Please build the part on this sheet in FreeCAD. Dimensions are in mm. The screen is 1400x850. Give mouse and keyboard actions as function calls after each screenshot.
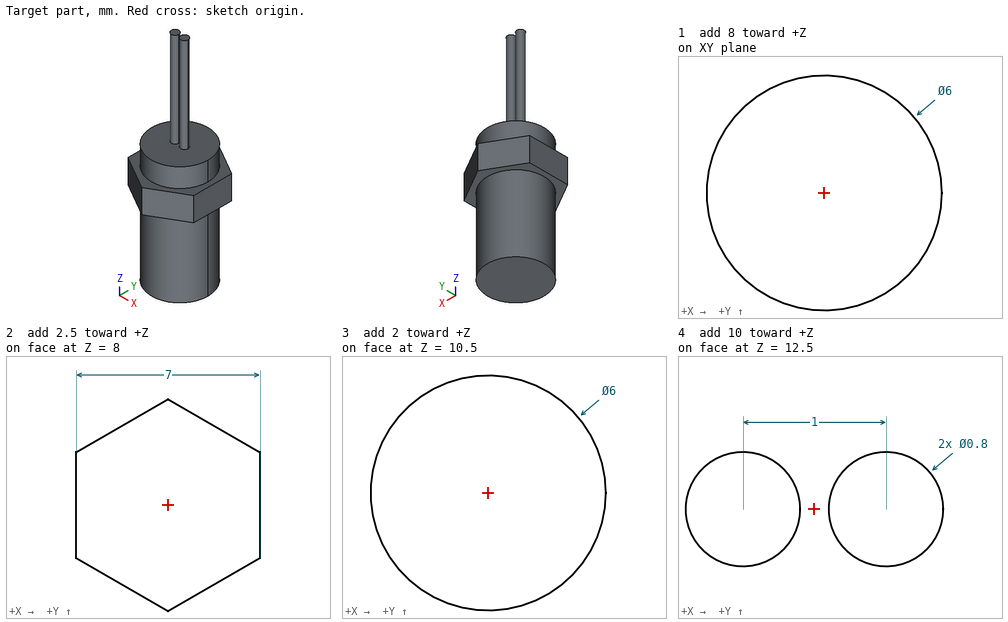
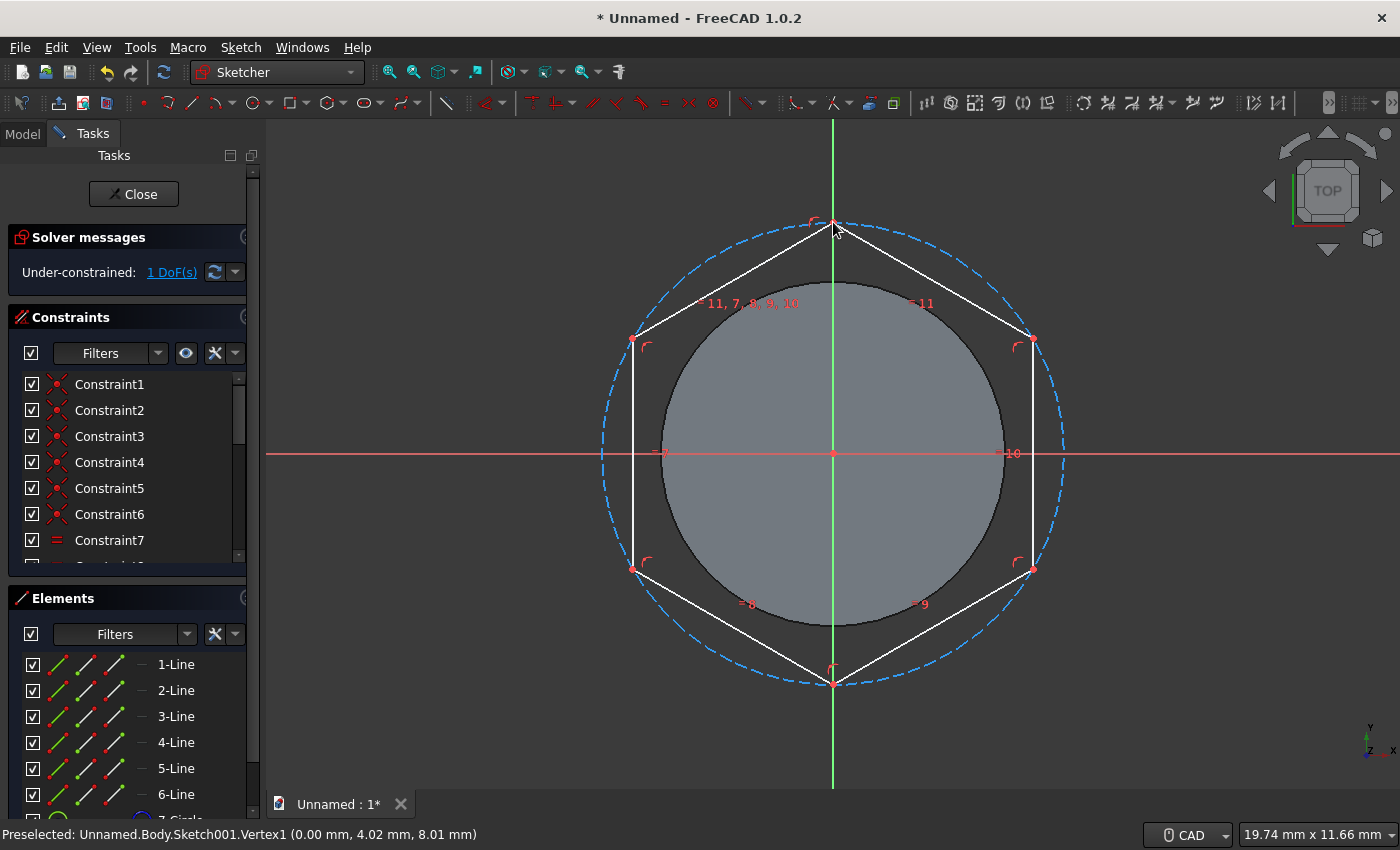
click(633, 339)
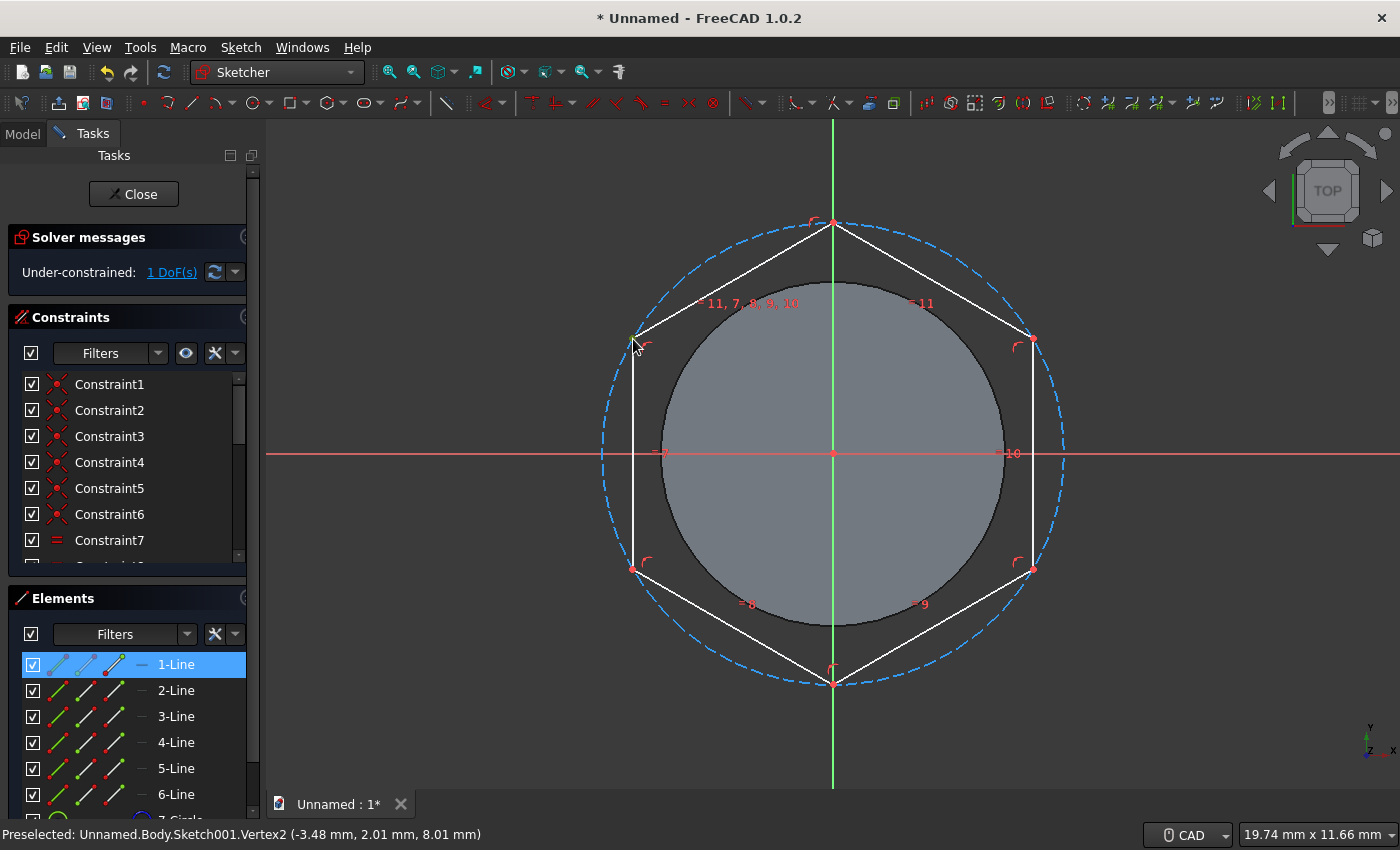
click(1033, 569)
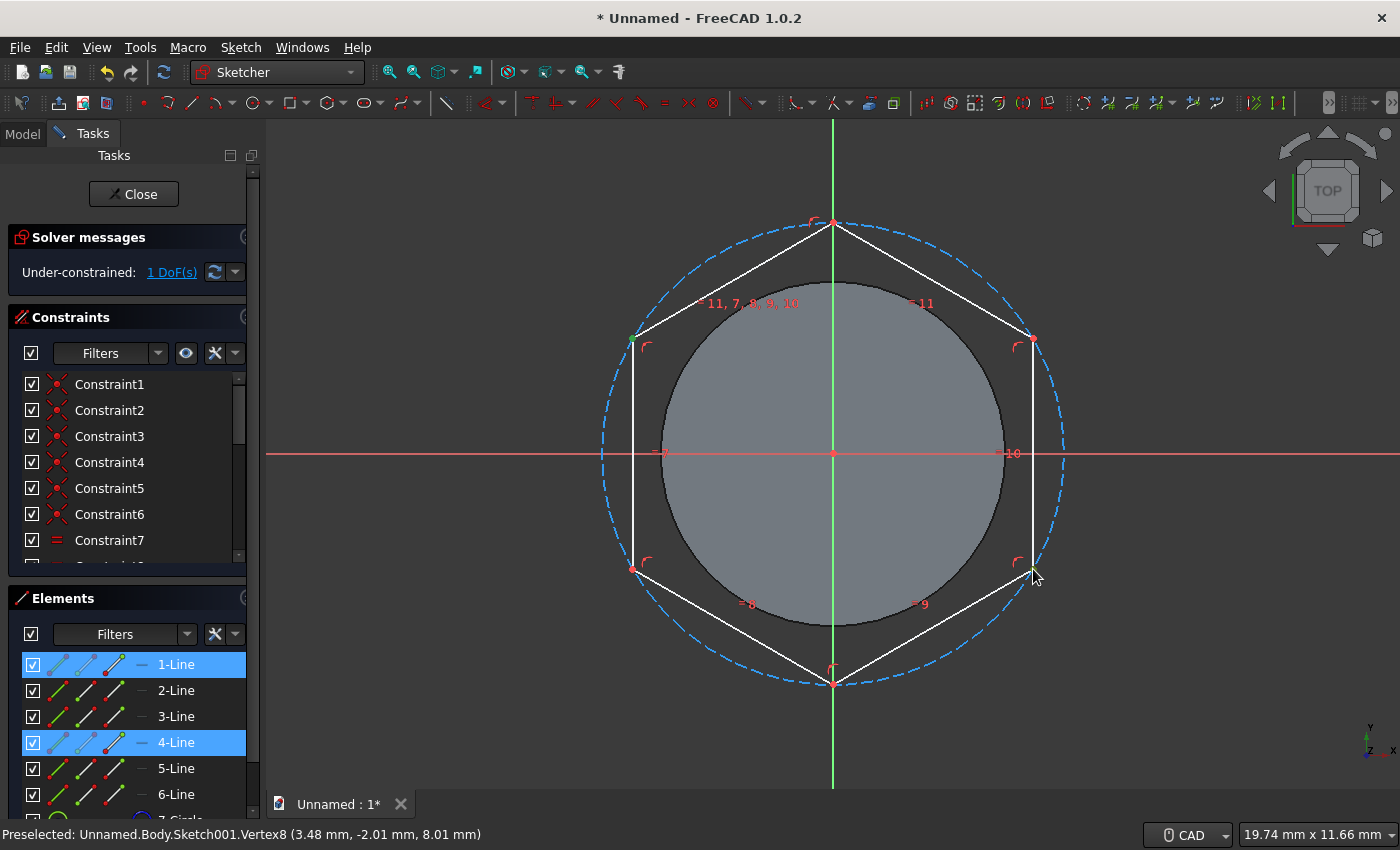
key(l)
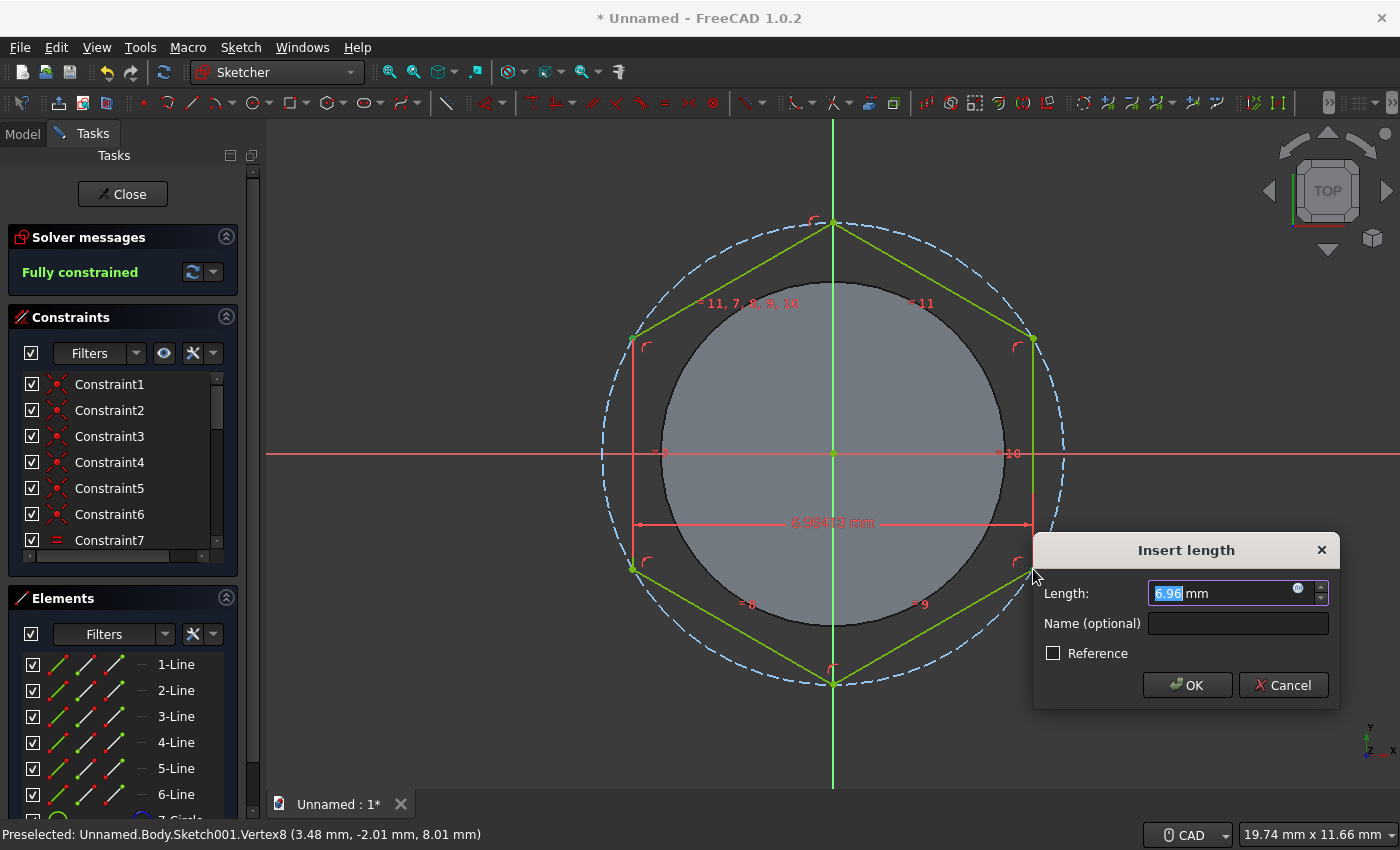
text(7)
key(Return)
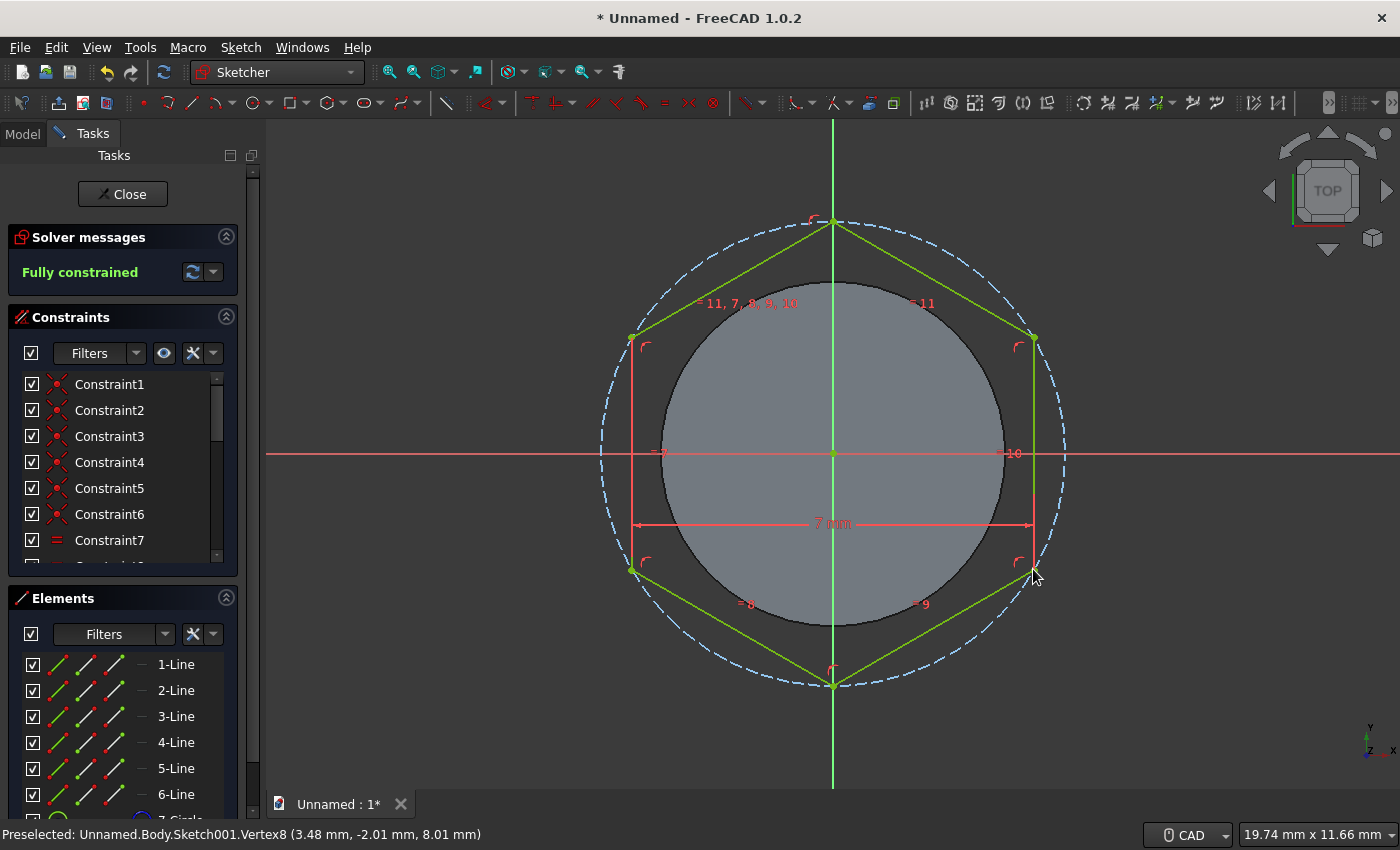
click(123, 194)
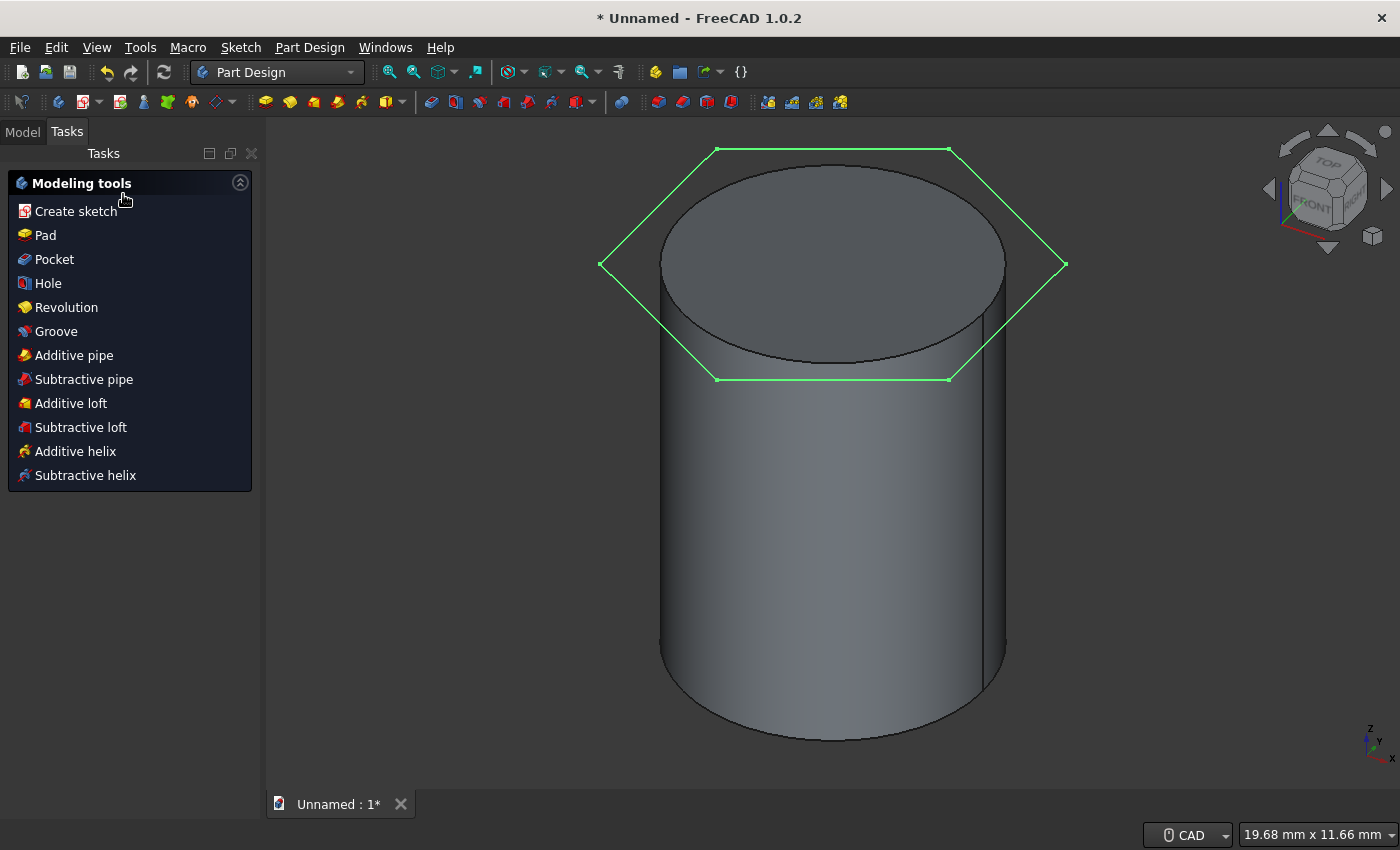
click(266, 102)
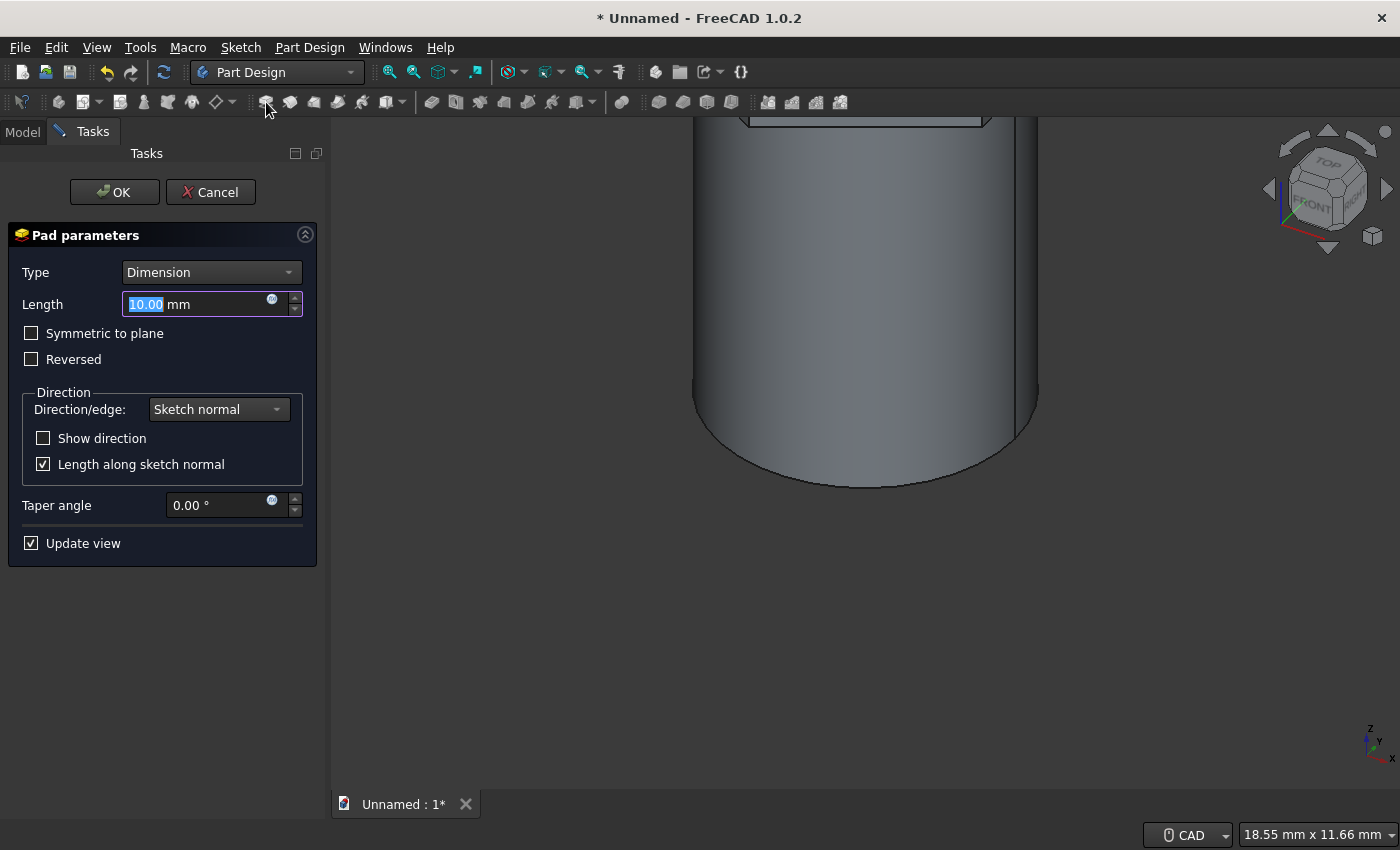
text(2.5)
key(Tab)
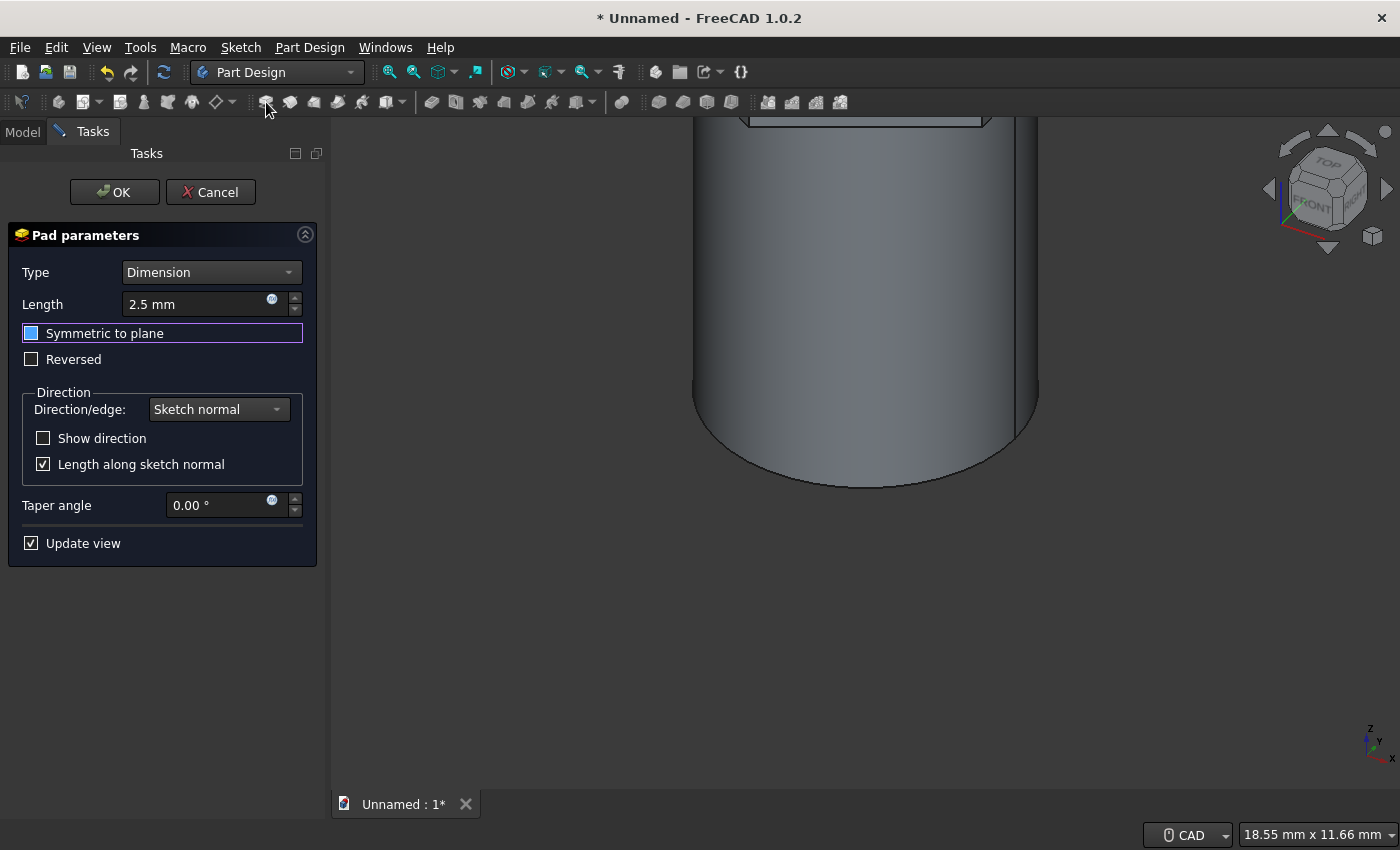
click(115, 192)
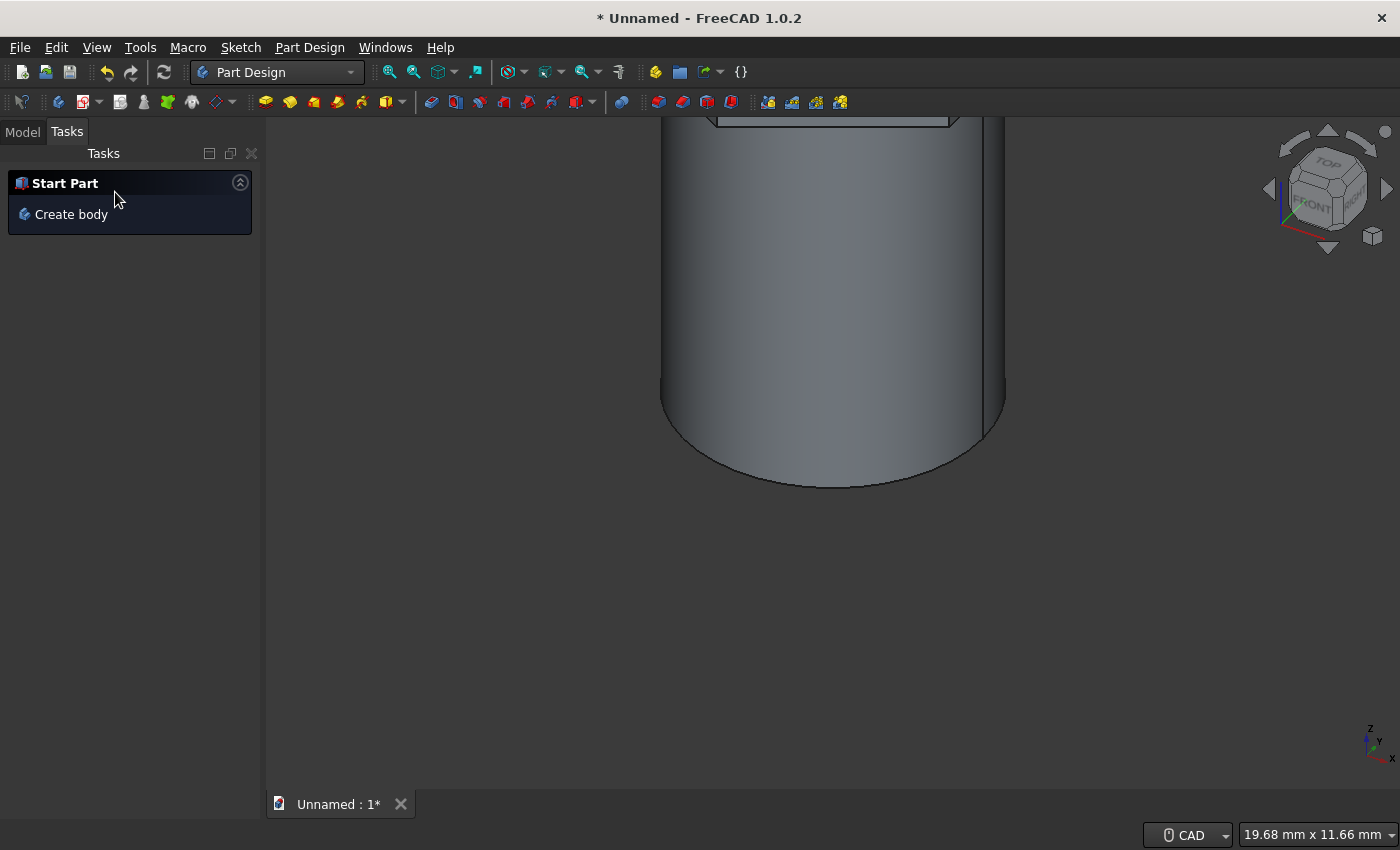
click(390, 72)